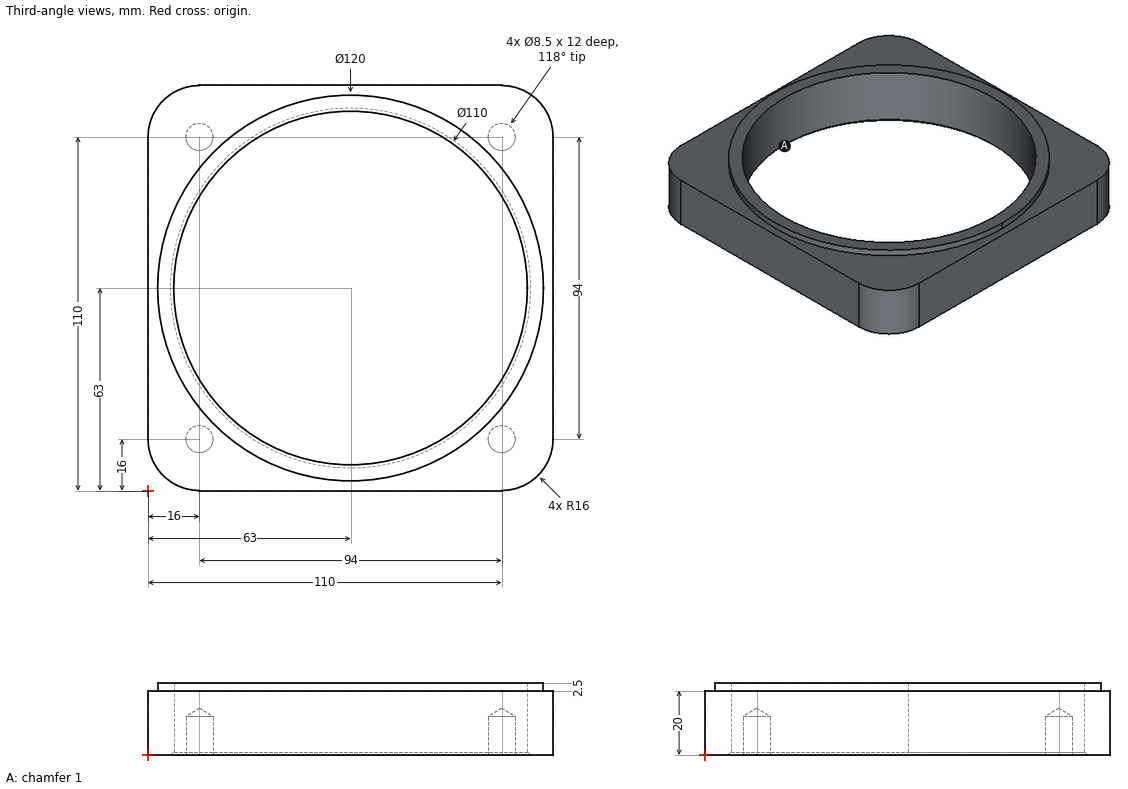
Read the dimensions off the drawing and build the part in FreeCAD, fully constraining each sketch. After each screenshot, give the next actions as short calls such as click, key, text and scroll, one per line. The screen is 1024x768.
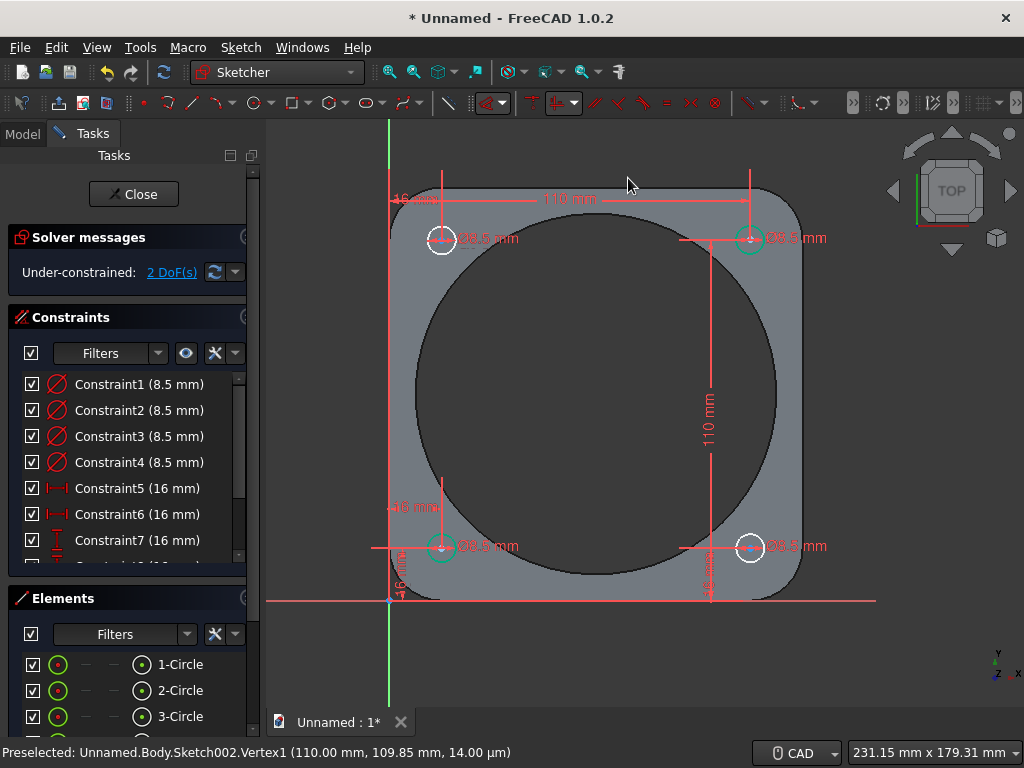
click(442, 241)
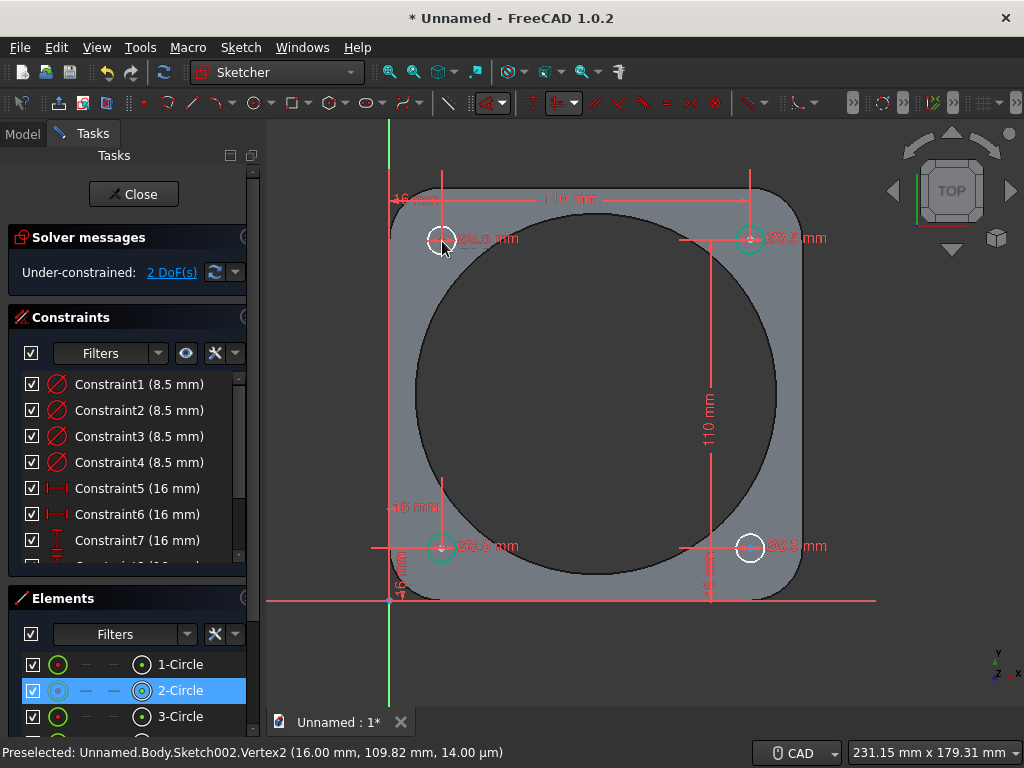
key(i)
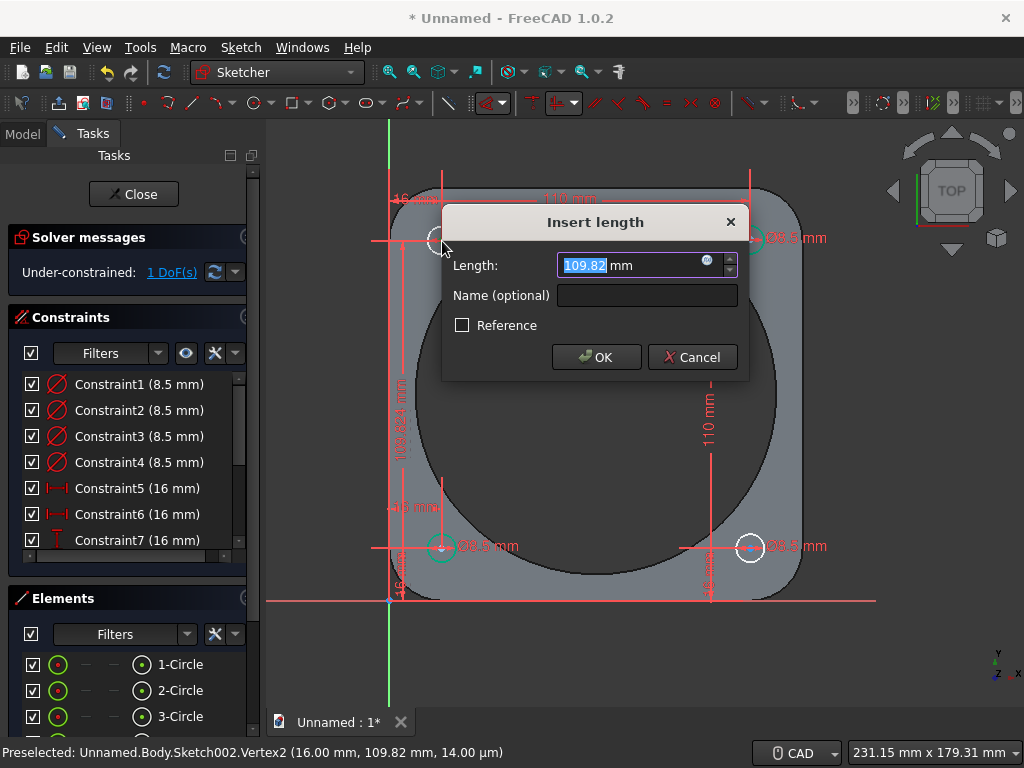
text(110)
key(Return)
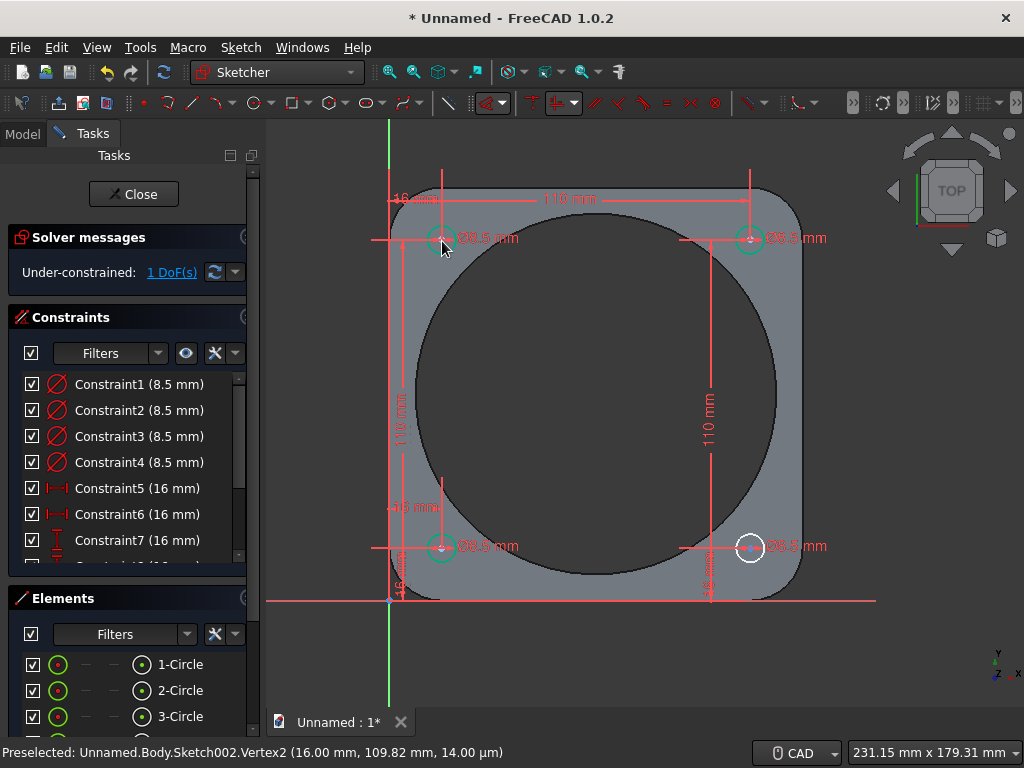
click(750, 548)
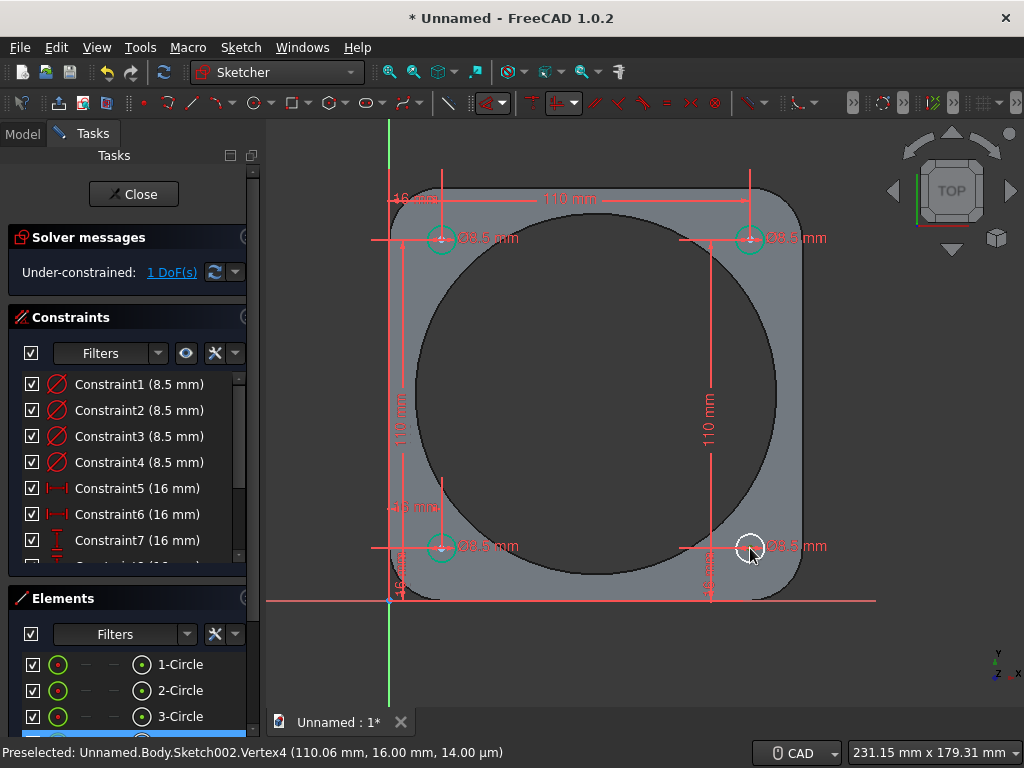
click(504, 104)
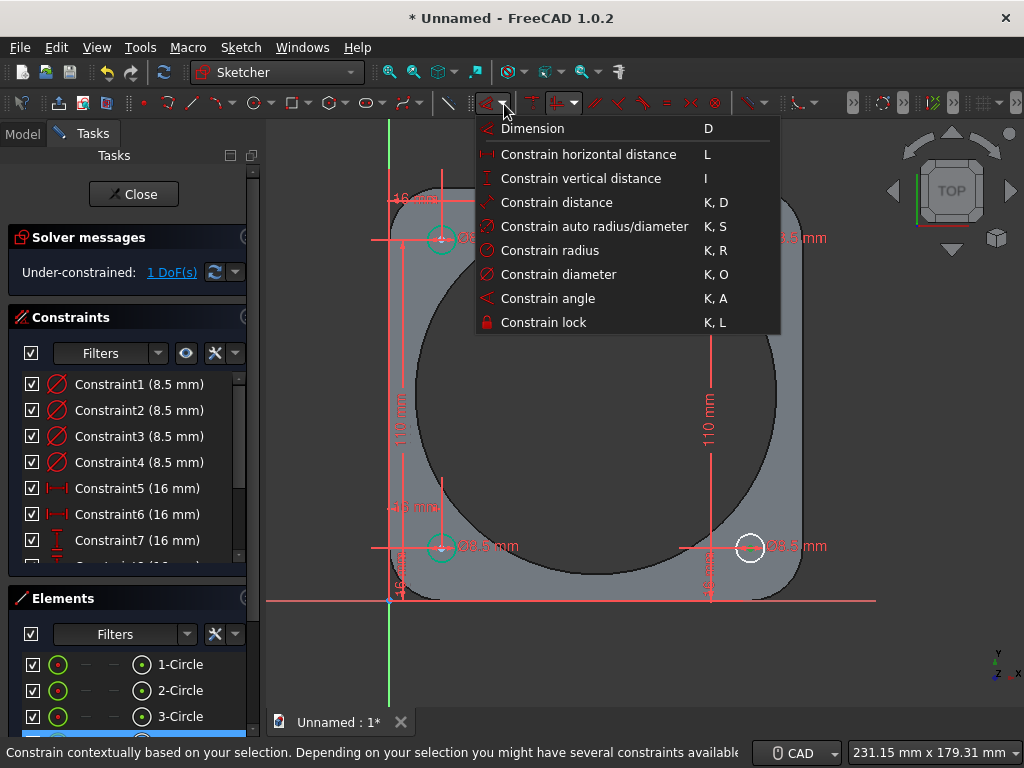
click(628, 154)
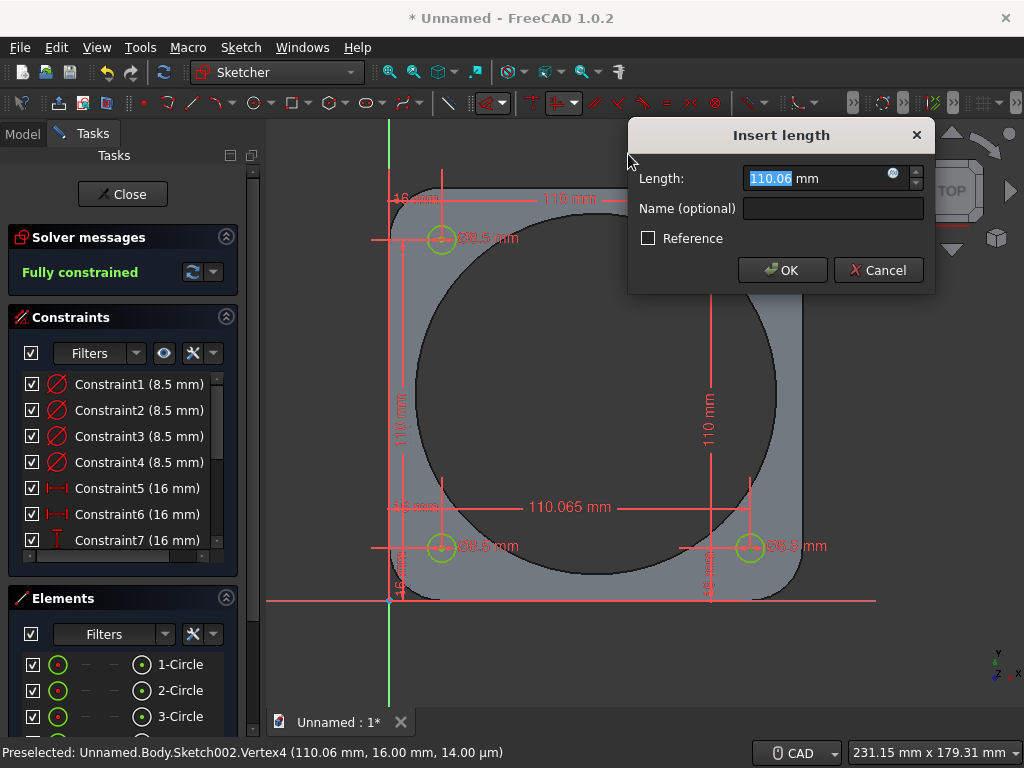
text(110)
key(Return)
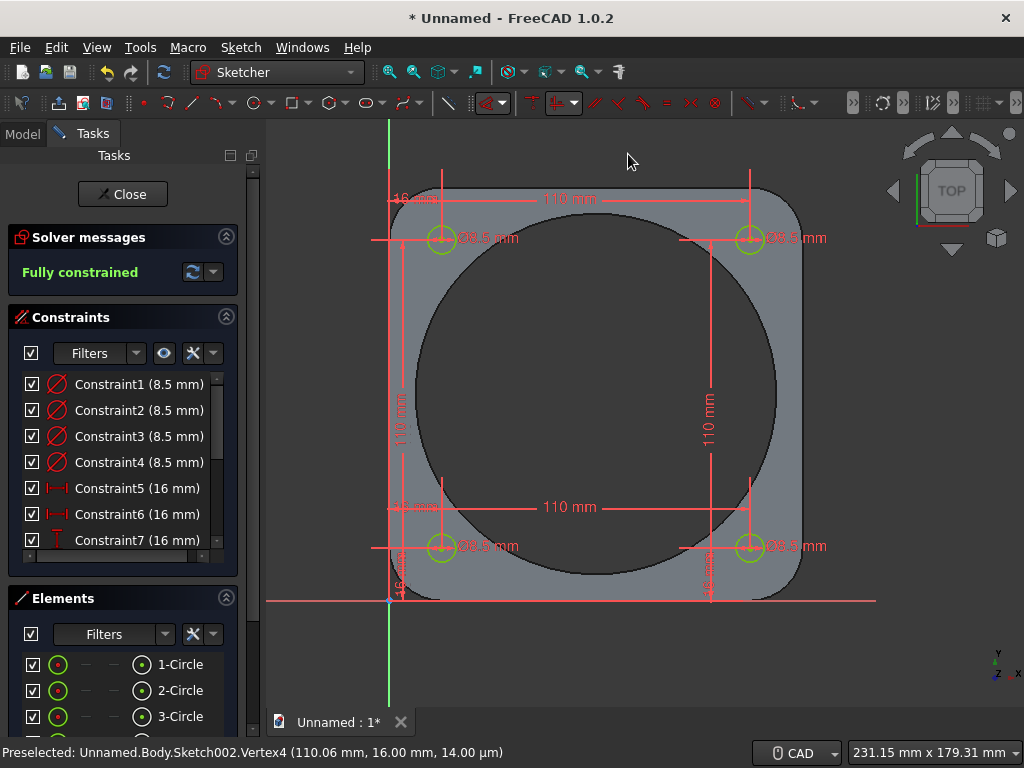
click(123, 194)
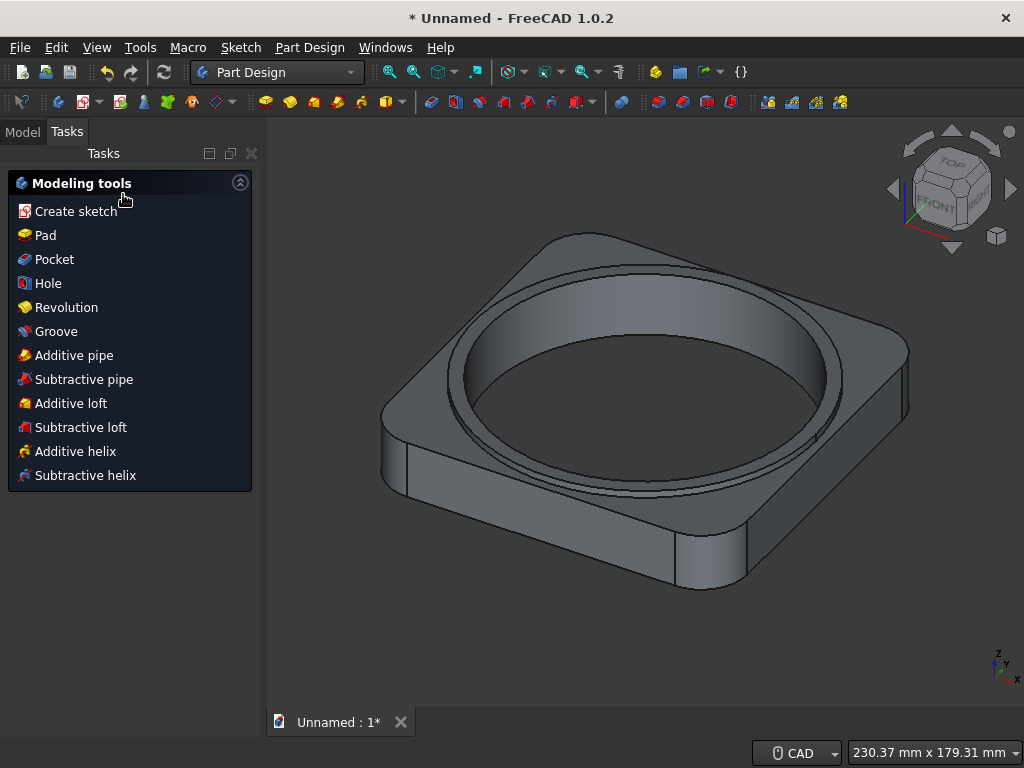
click(456, 102)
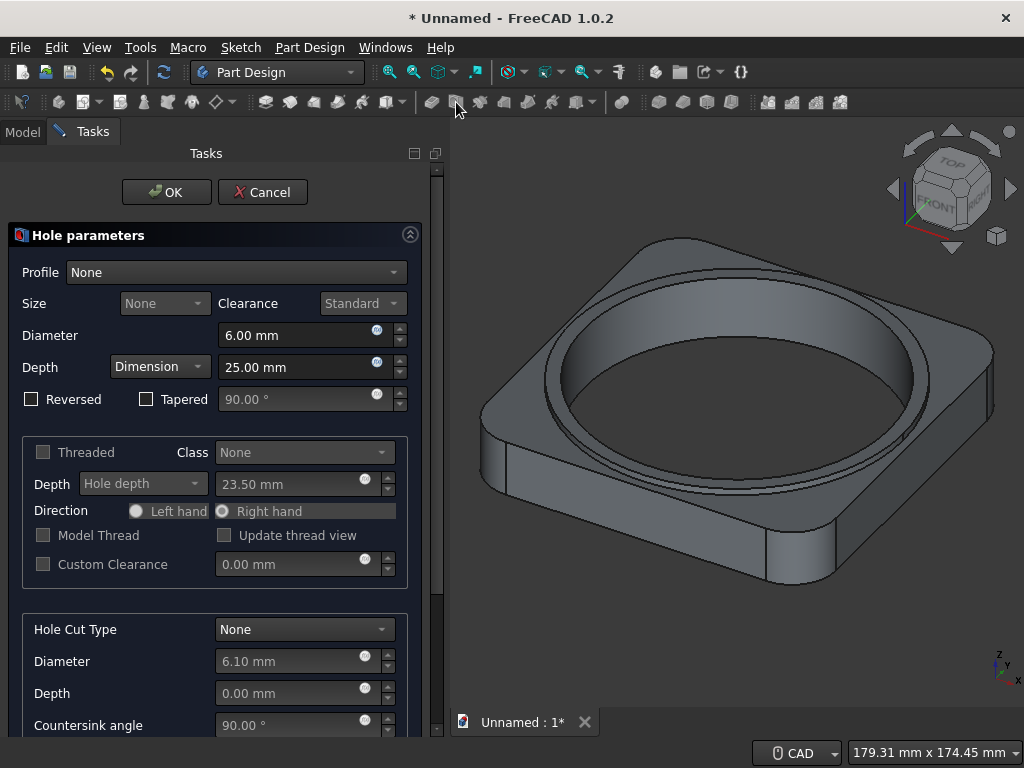
triple_click(305, 335)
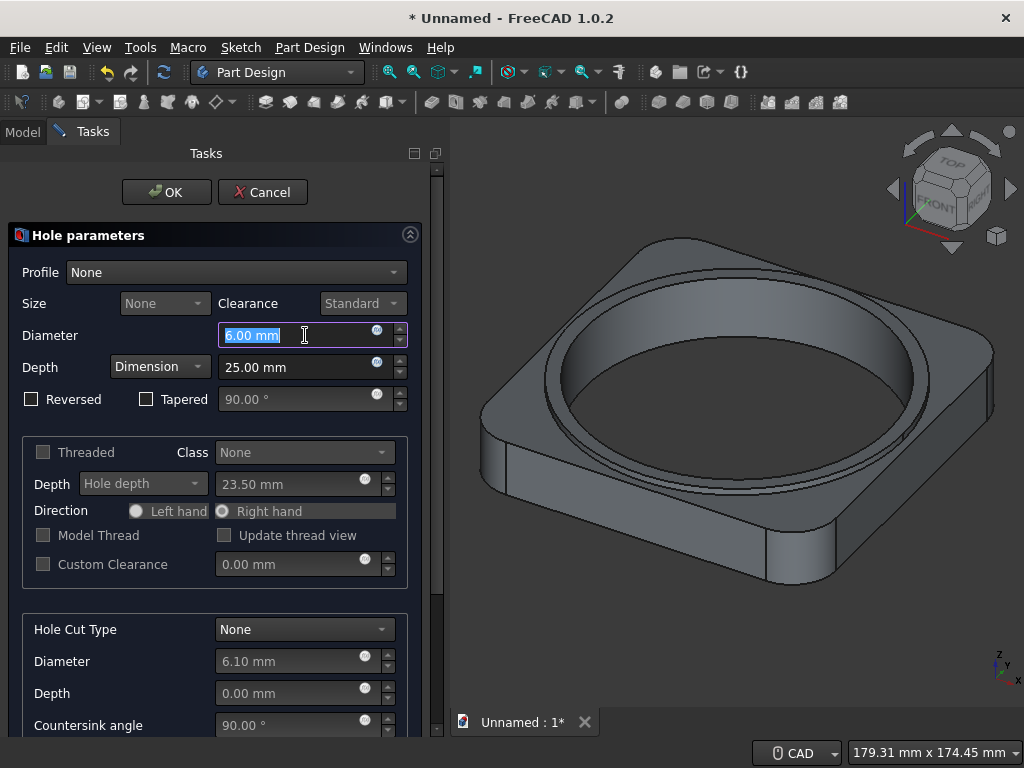
text(8.5)
key(Tab)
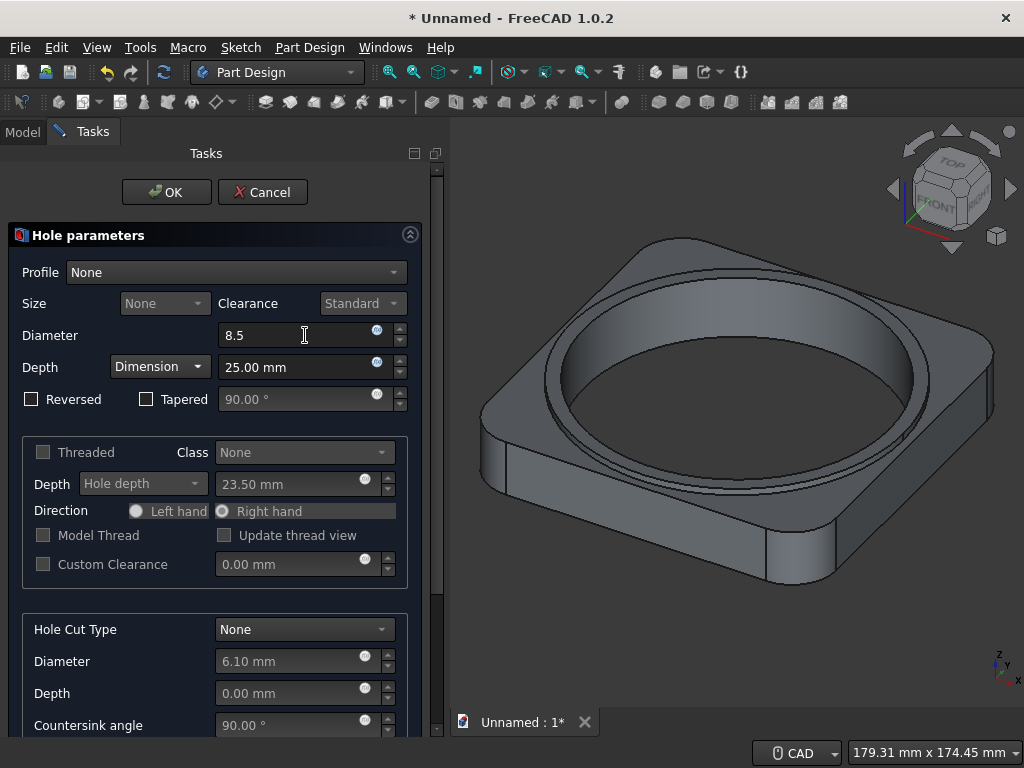
triple_click(305, 367)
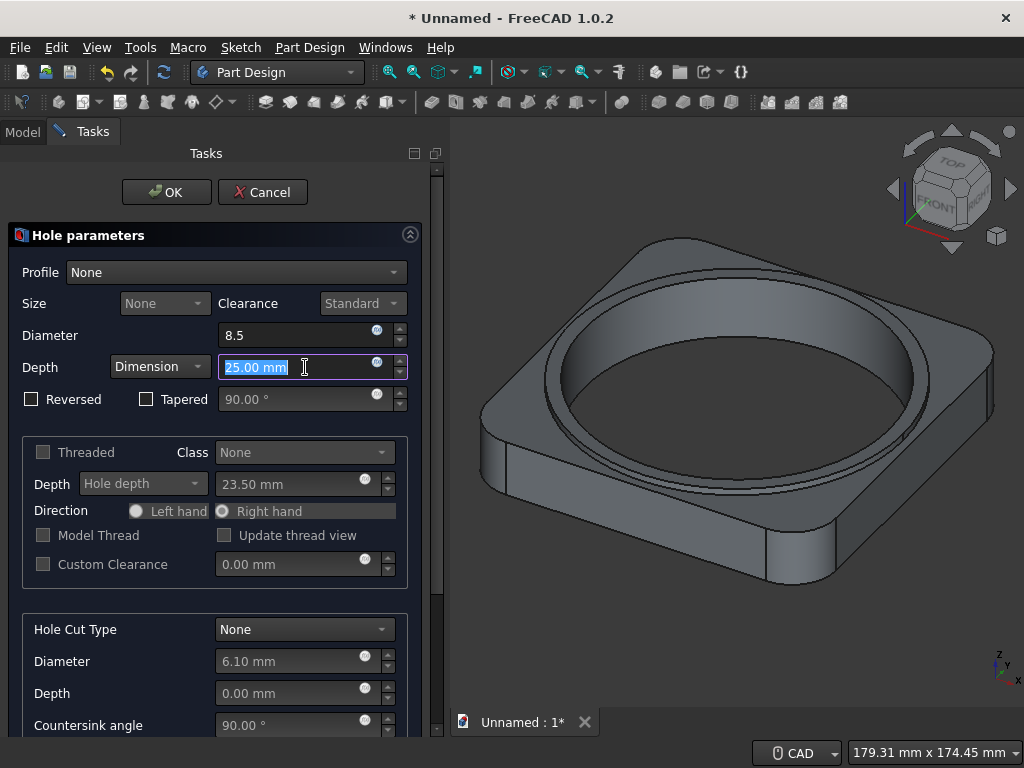
text(12)
key(Tab)